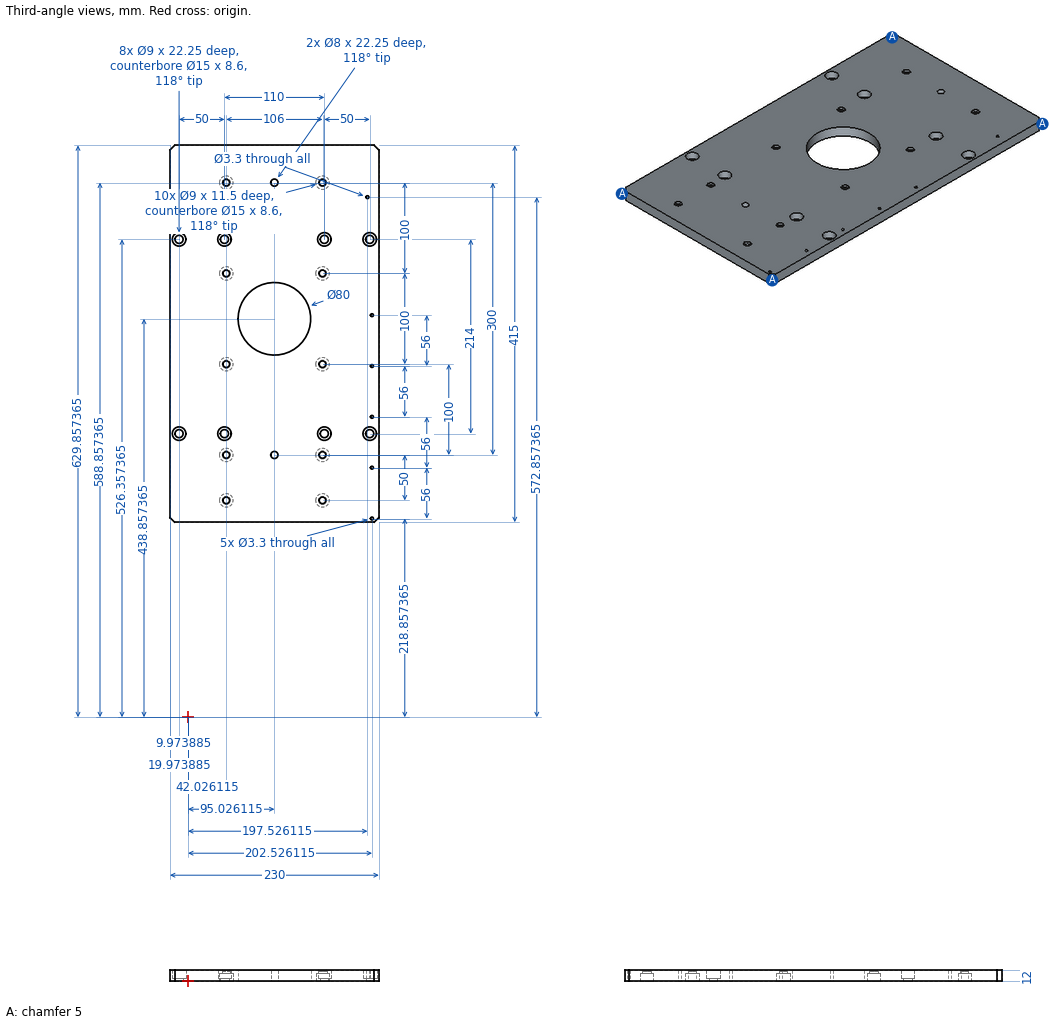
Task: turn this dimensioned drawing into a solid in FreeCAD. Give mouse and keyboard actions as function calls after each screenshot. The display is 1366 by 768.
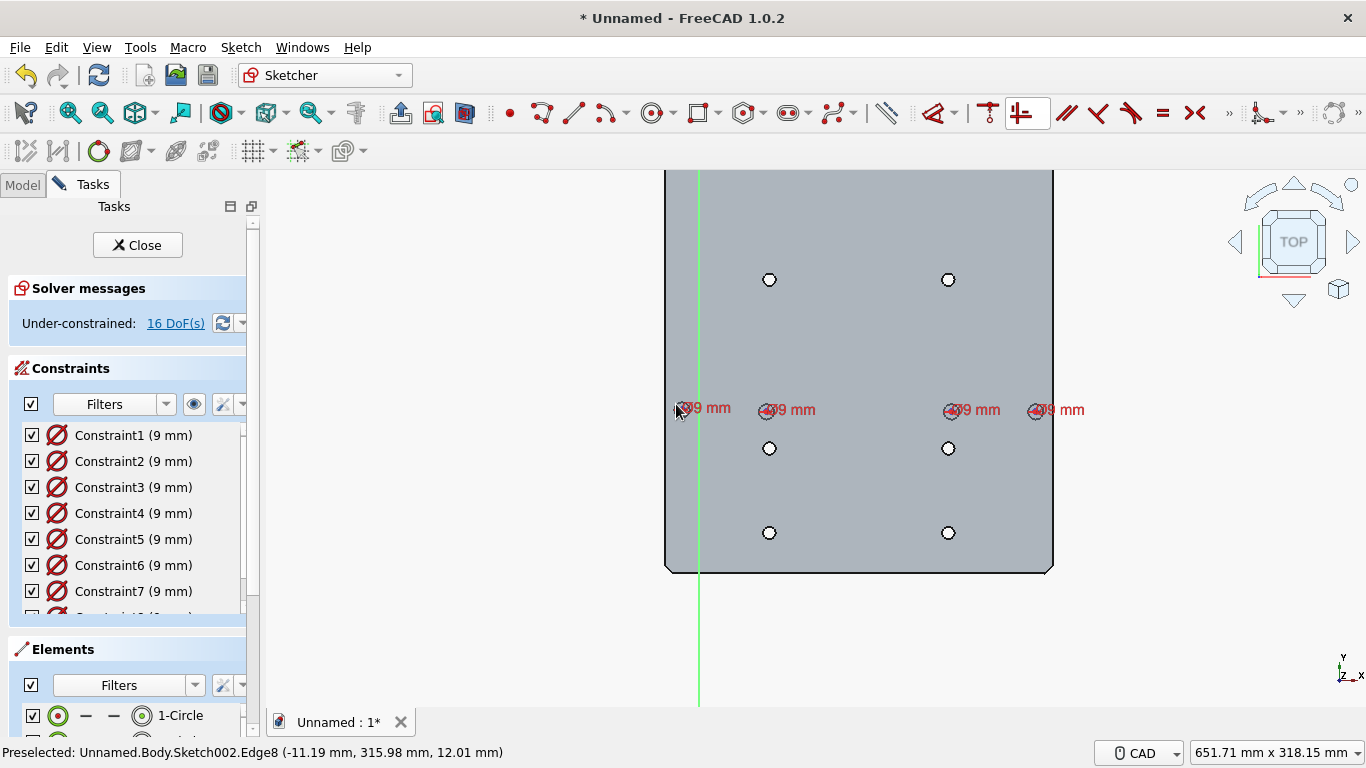
scroll(683, 410, down, 5)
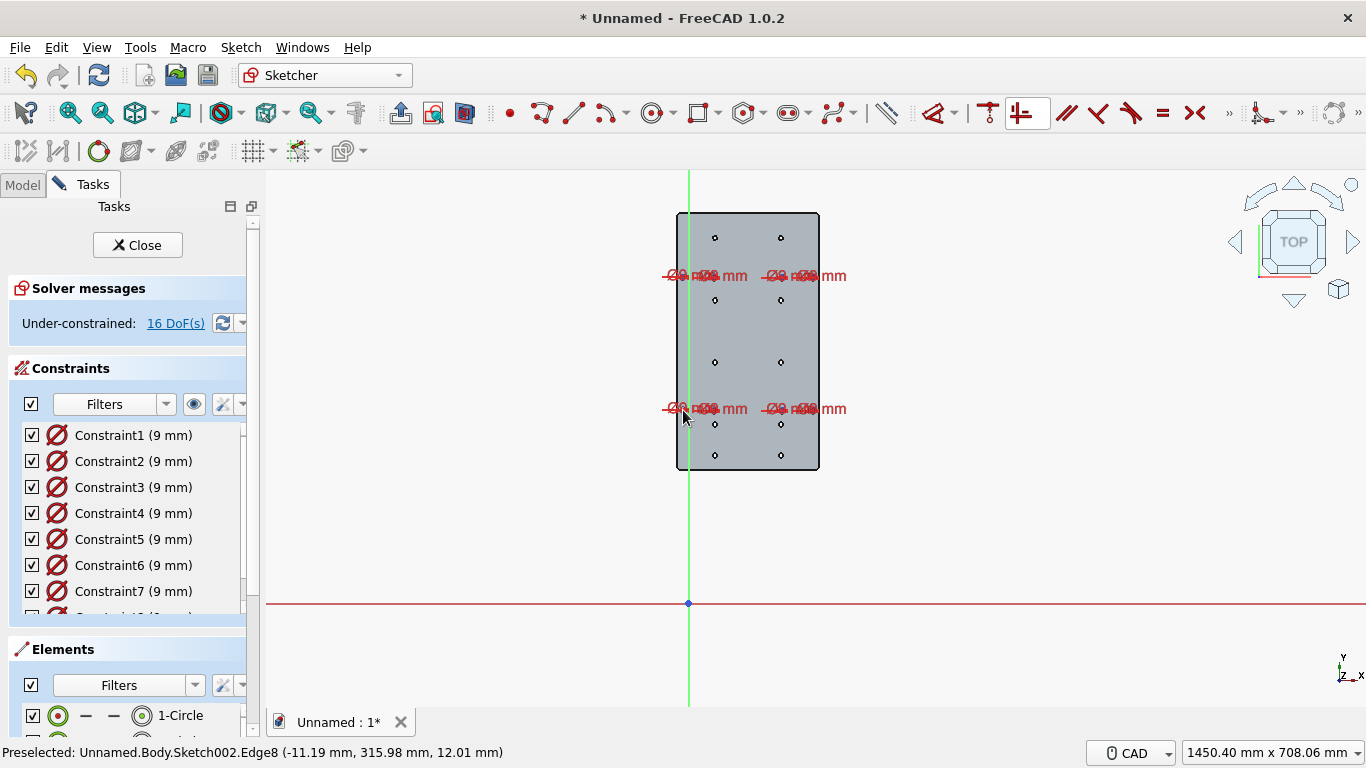
click(683, 277)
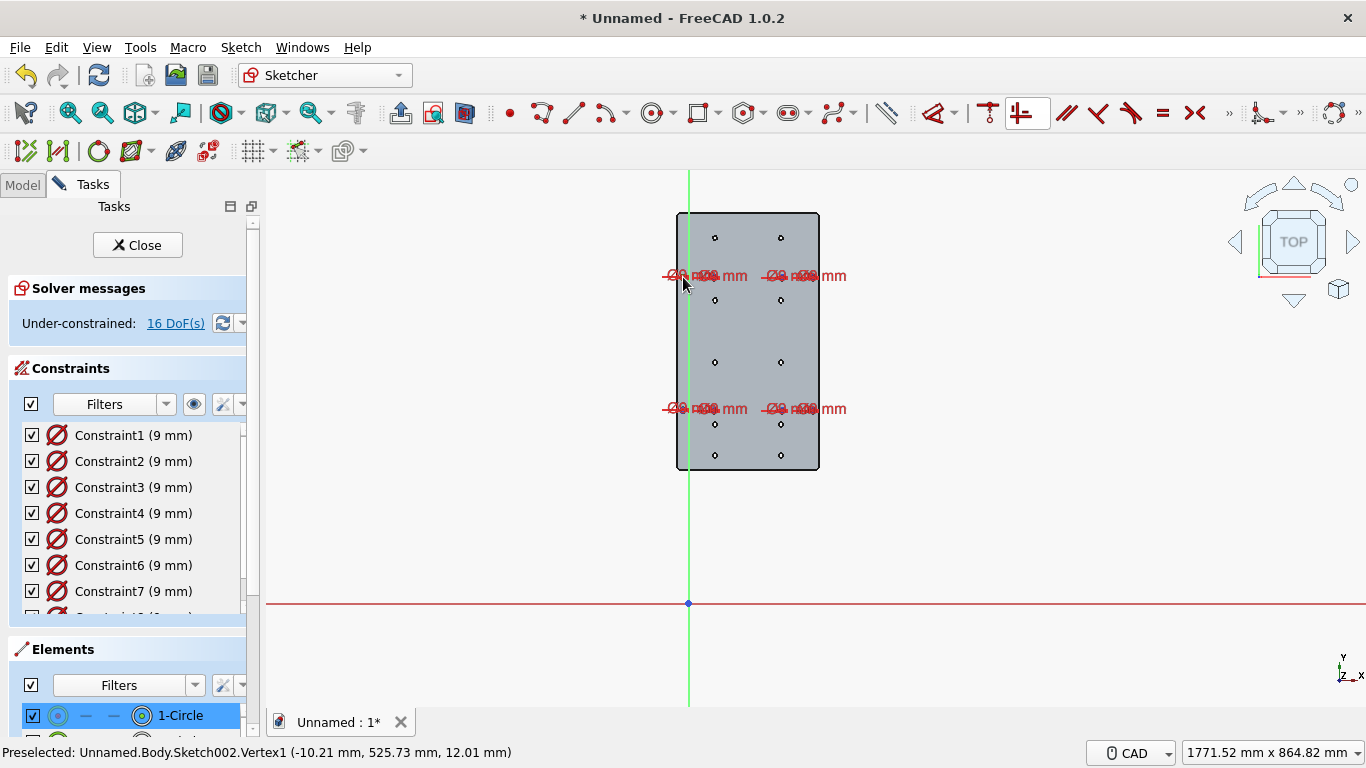
click(714, 278)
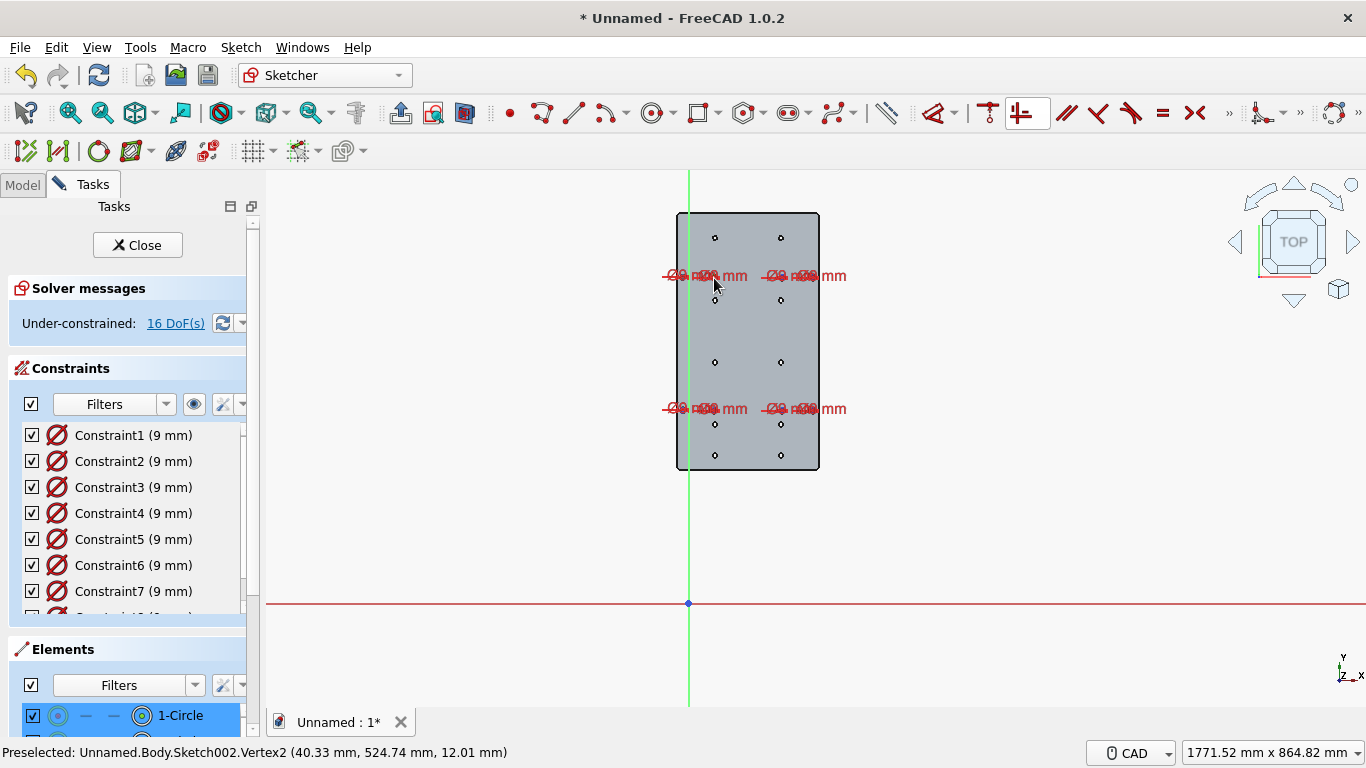
click(1044, 114)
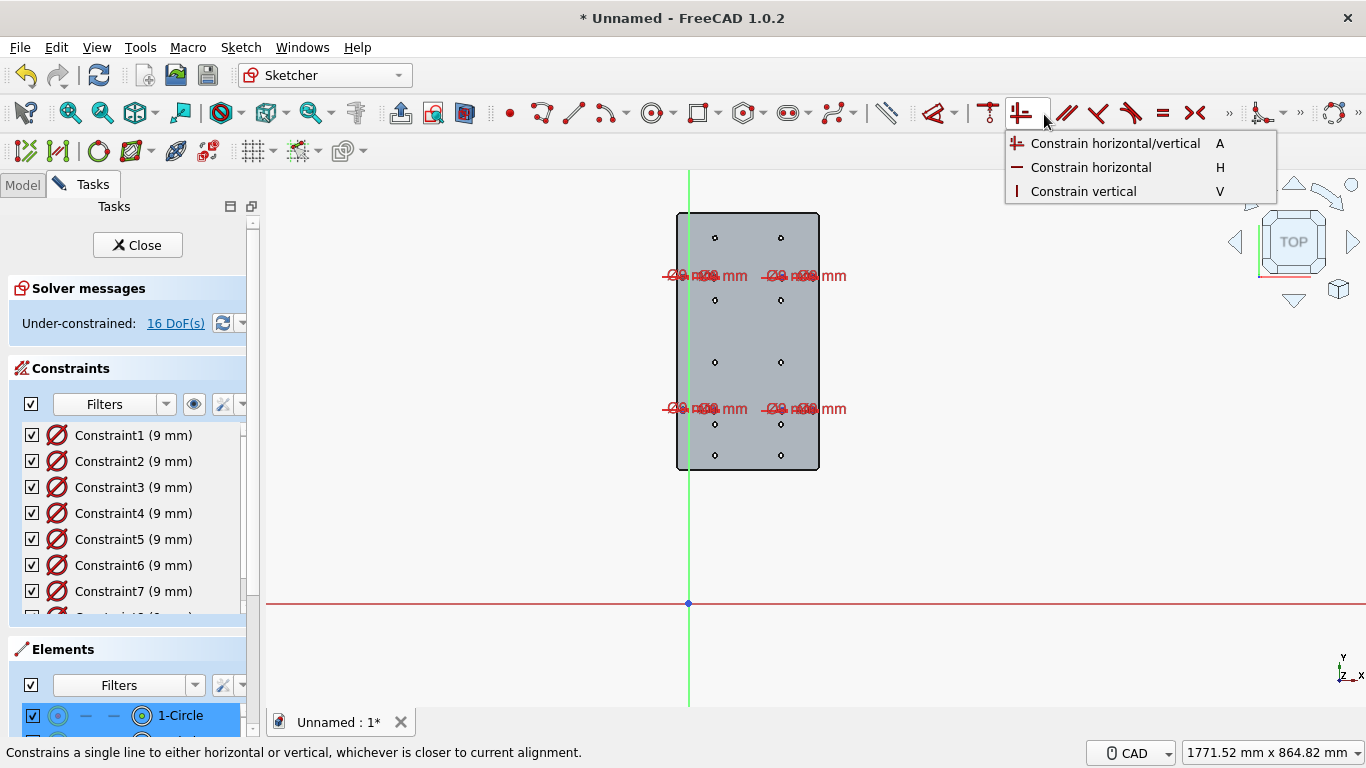
click(1141, 167)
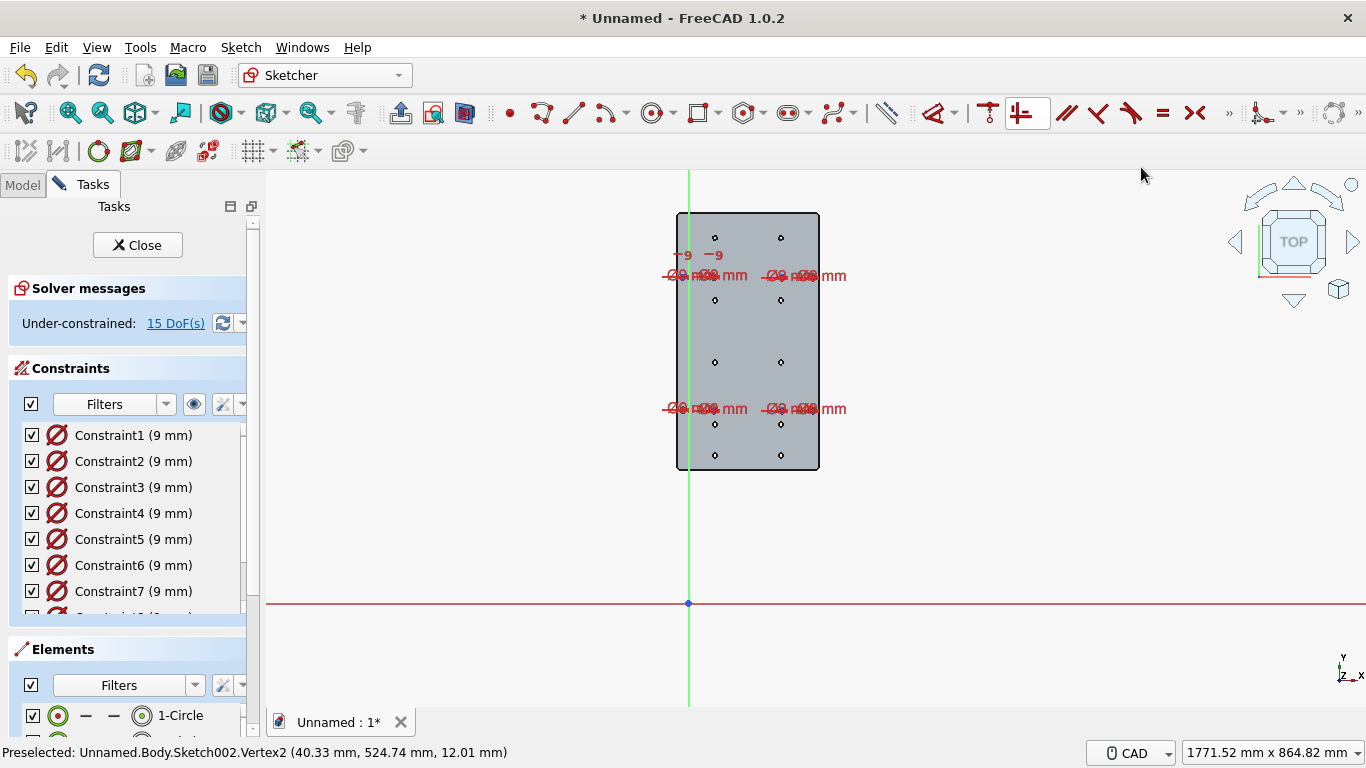
click(714, 277)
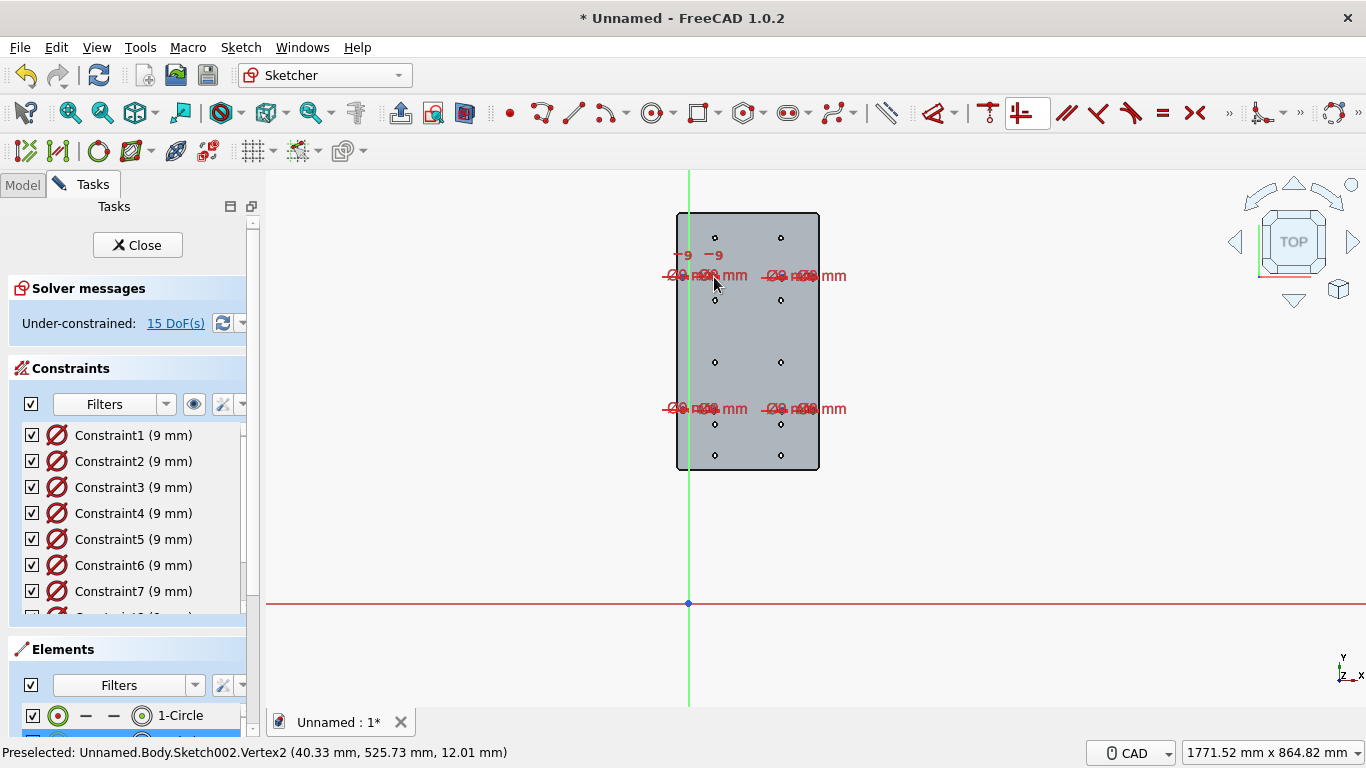
click(782, 278)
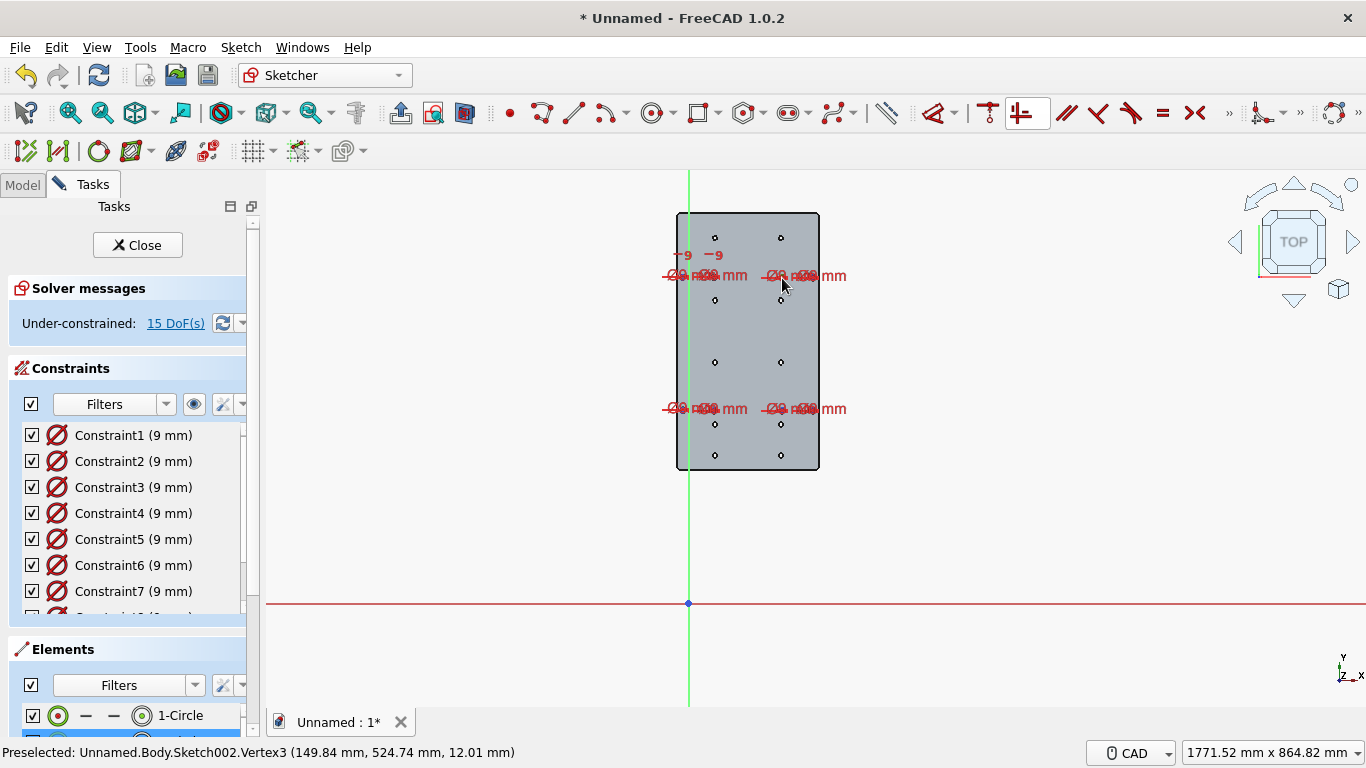
key(h)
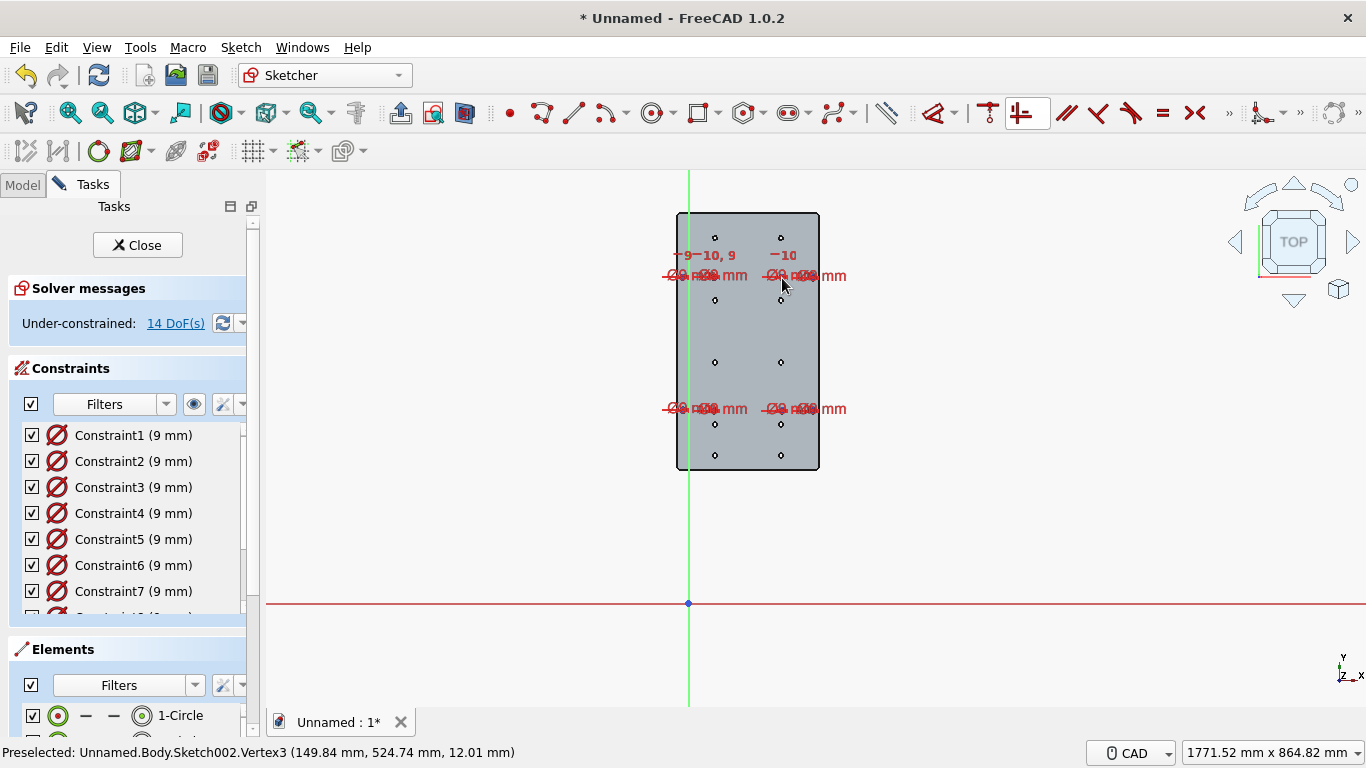
click(782, 277)